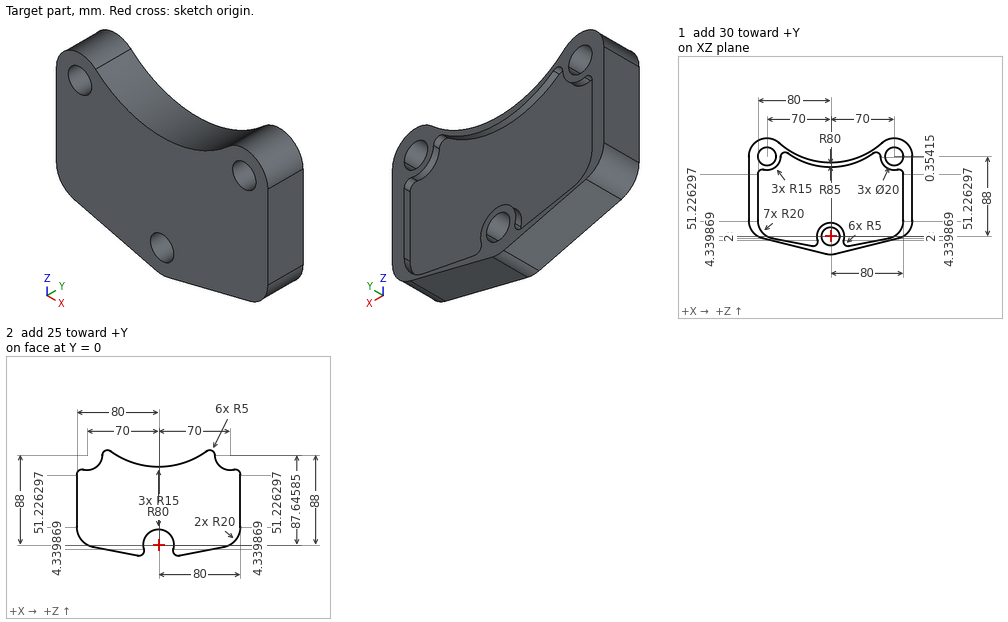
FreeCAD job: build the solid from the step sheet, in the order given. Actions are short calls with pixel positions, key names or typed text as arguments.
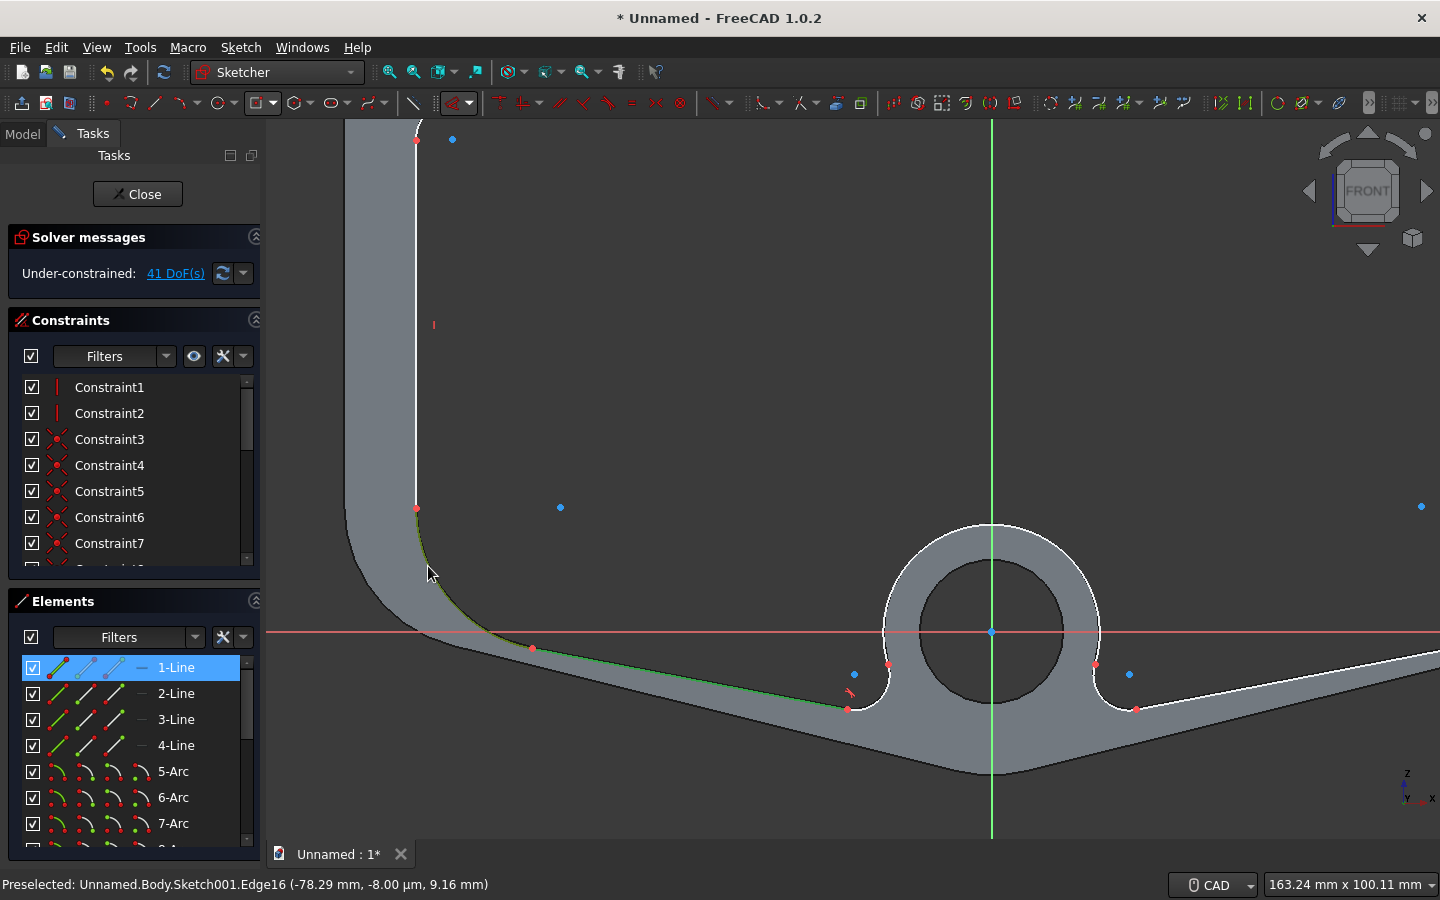
click(608, 104)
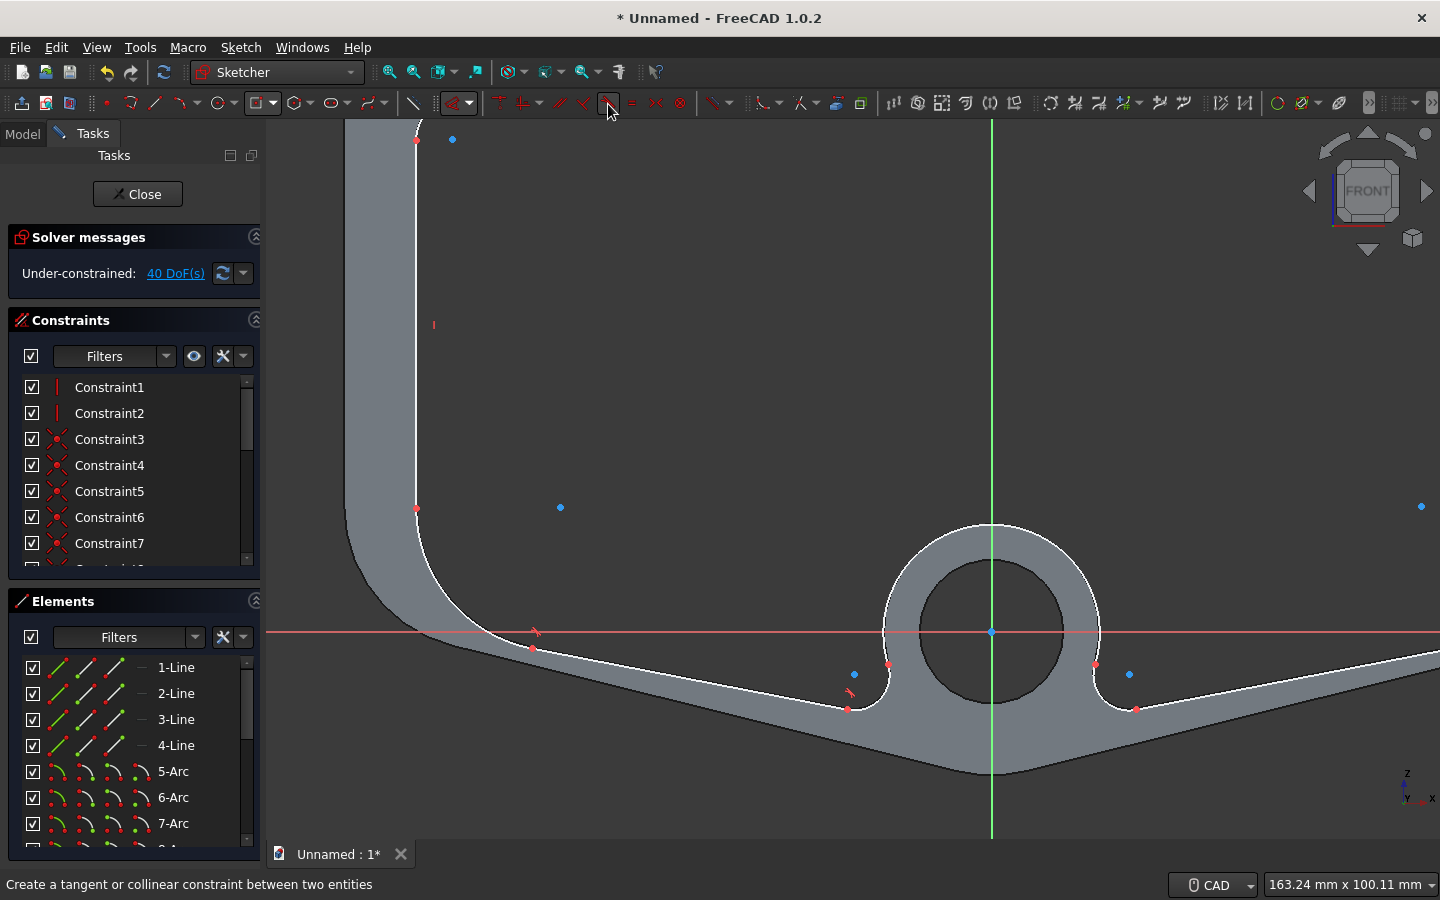
click(1231, 692)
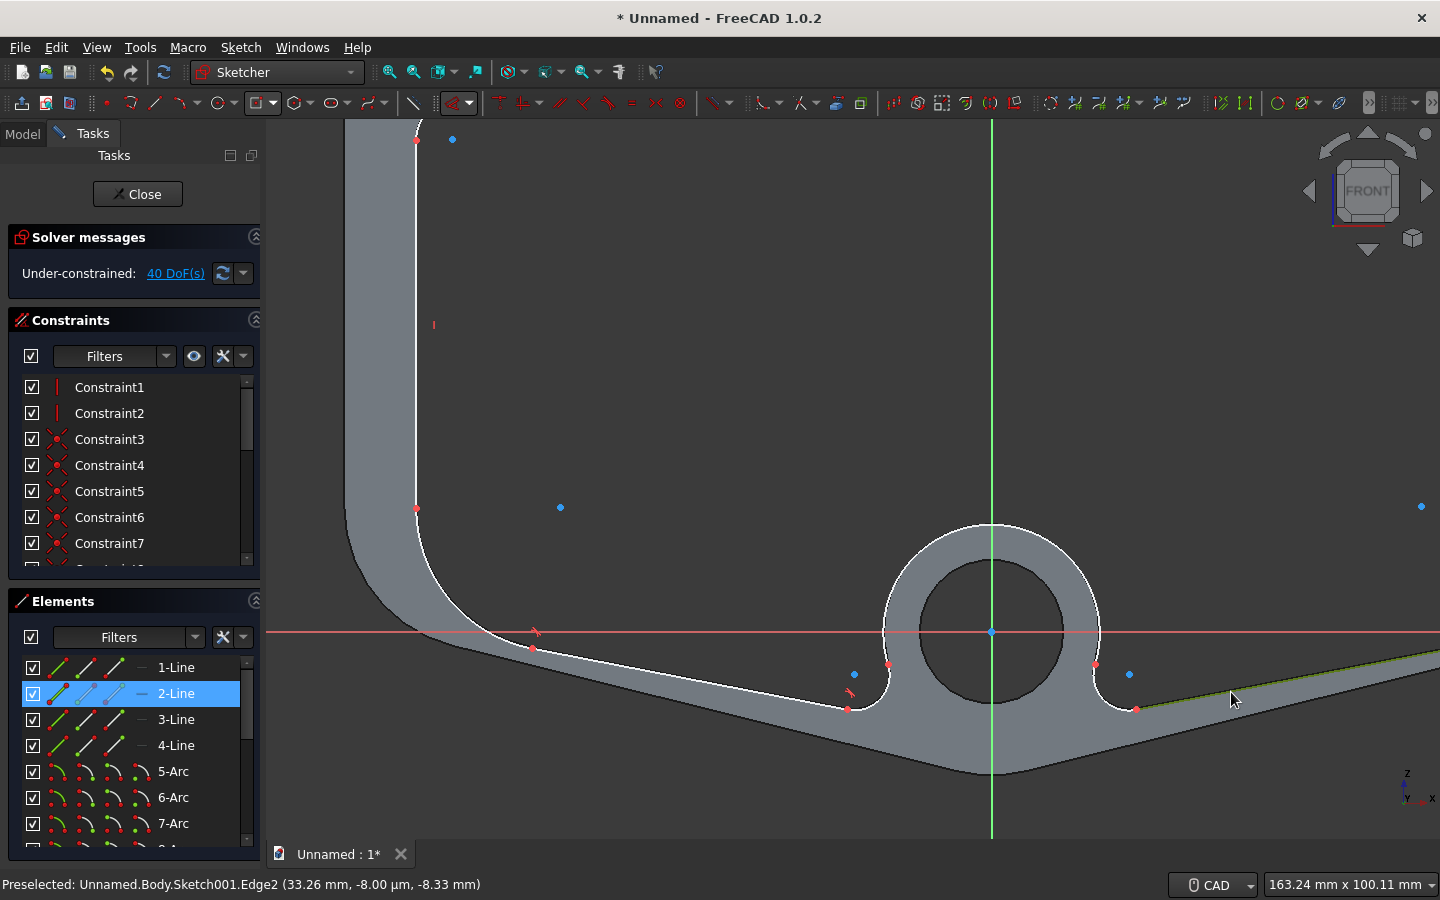
click(1095, 686)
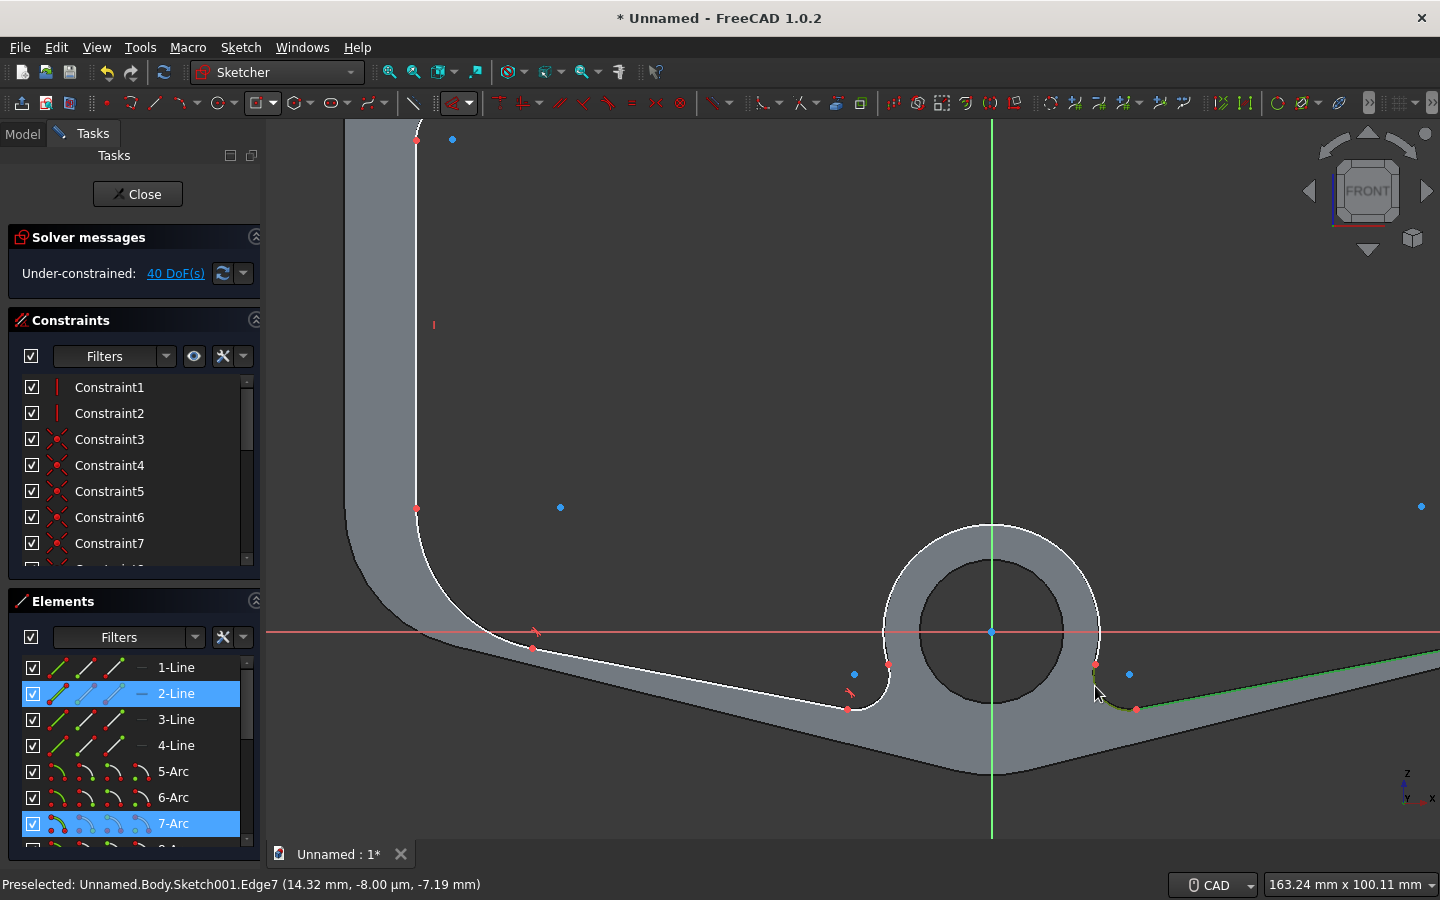
click(608, 104)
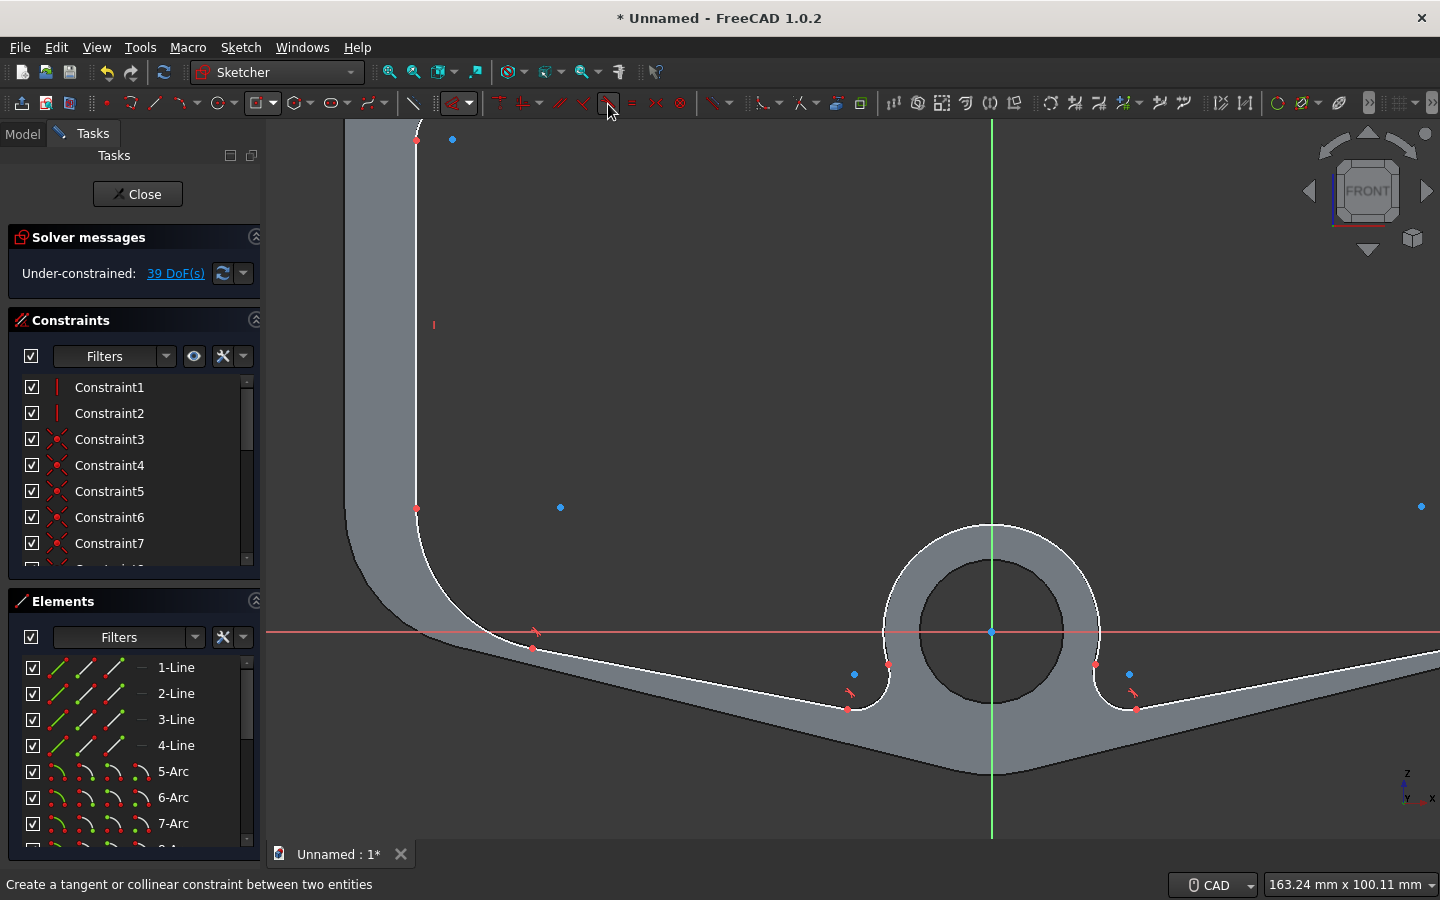
click(1231, 692)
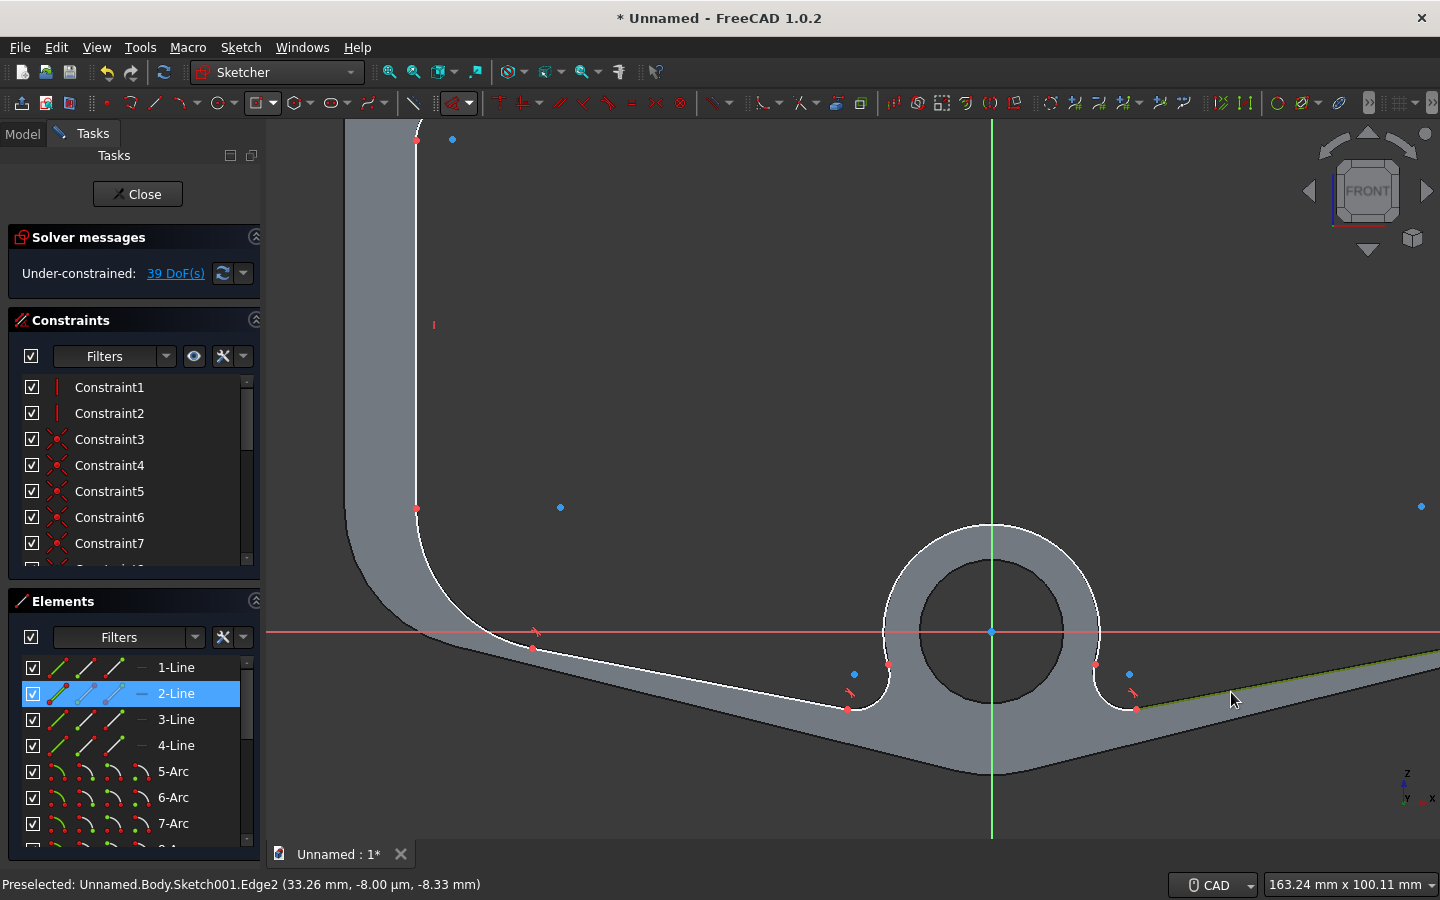
scroll(533, 649, down, 3)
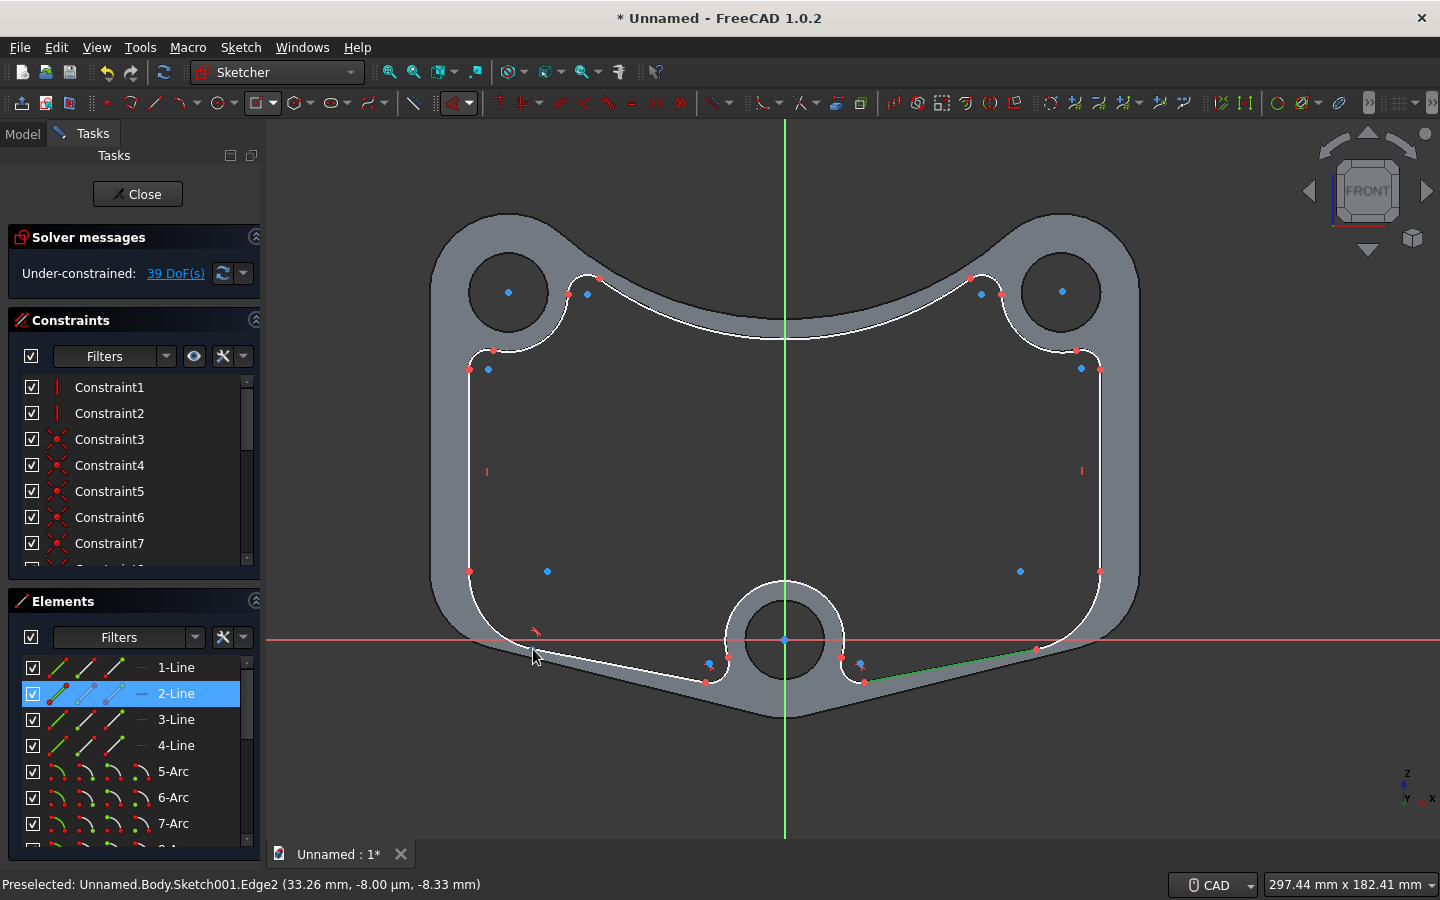
click(1094, 603)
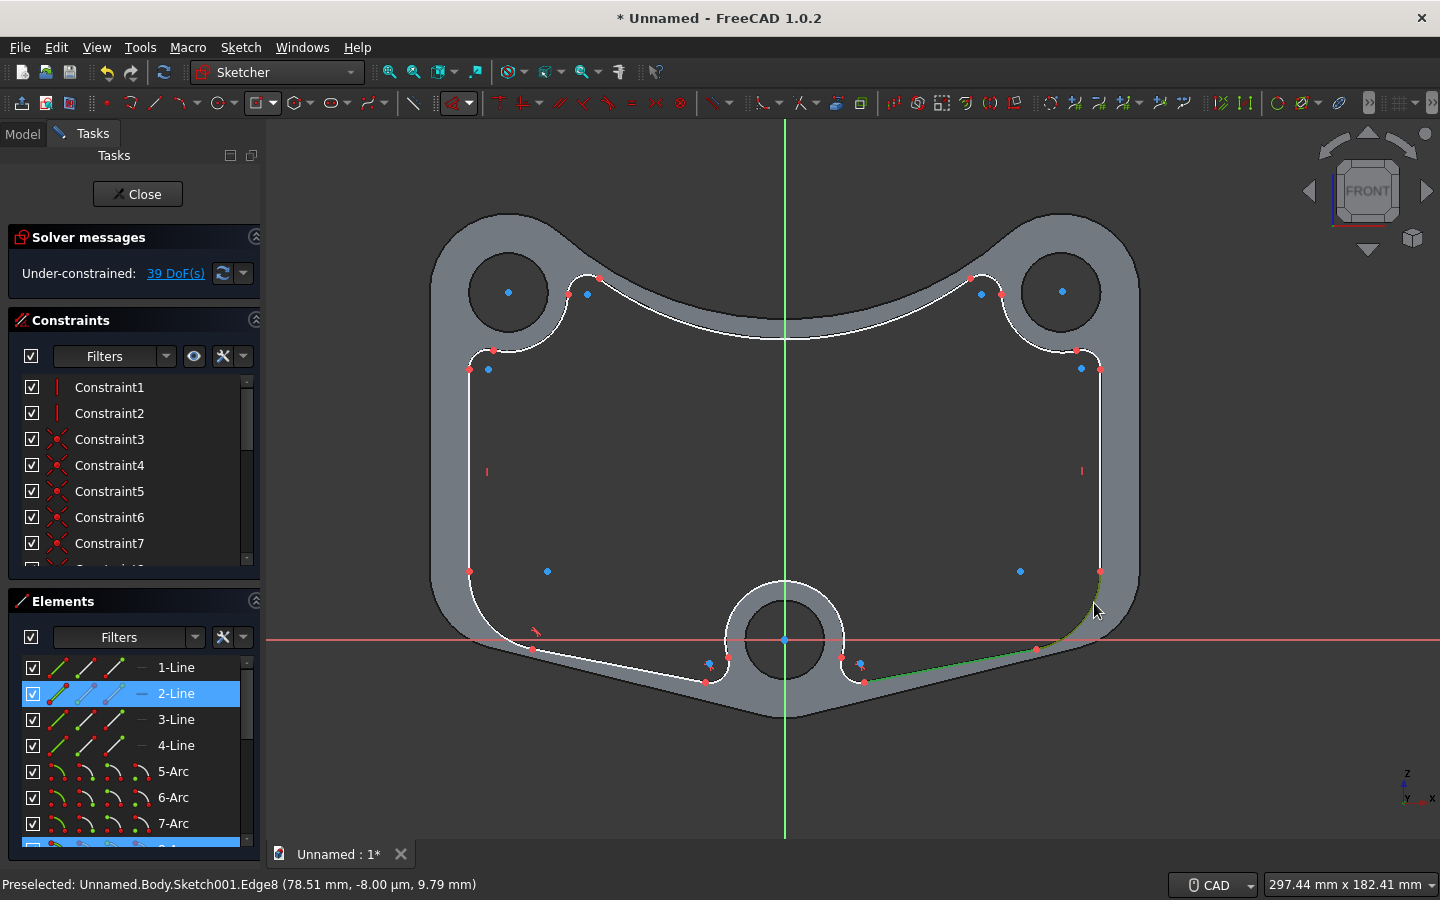
click(608, 104)